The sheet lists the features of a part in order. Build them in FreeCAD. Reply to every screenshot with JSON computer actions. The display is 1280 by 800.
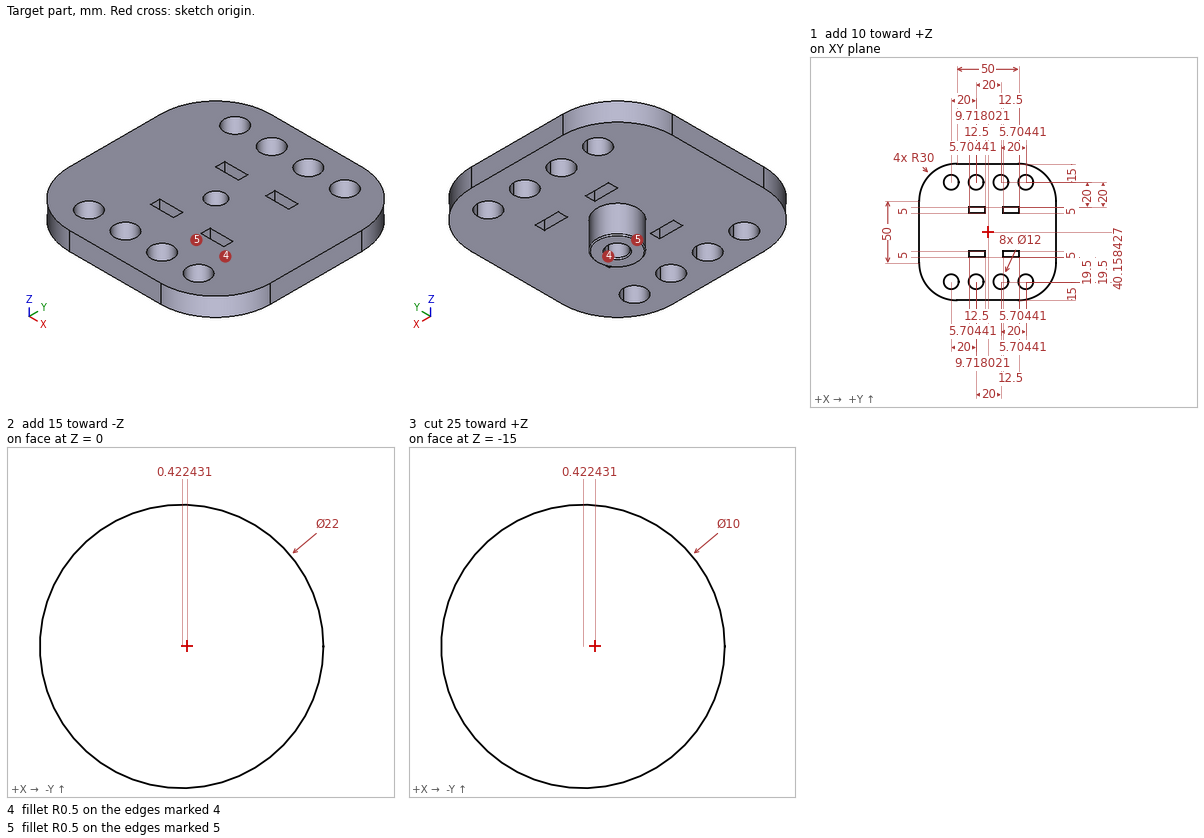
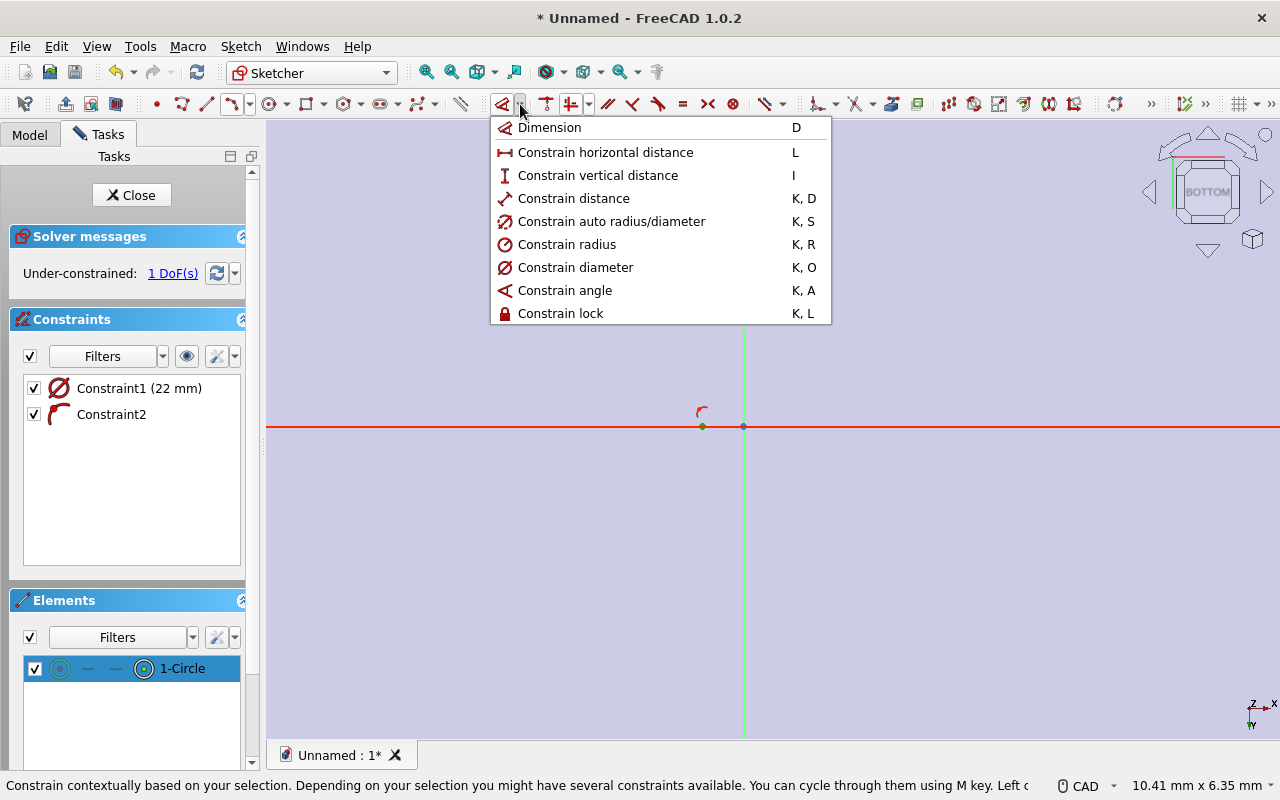
{"action": "left_click", "coordinate": [661, 152]}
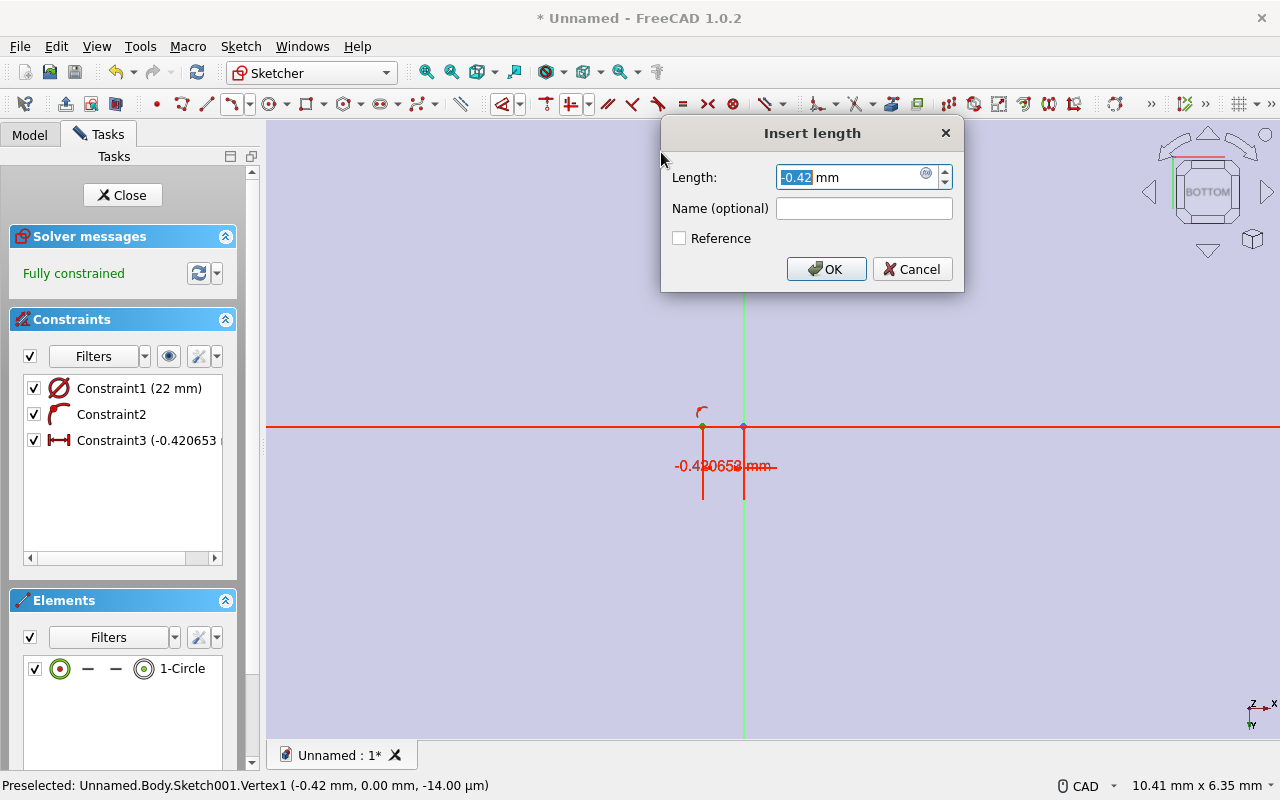
{"action": "type", "text": "-0.422431"}
{"action": "key", "text": "Return"}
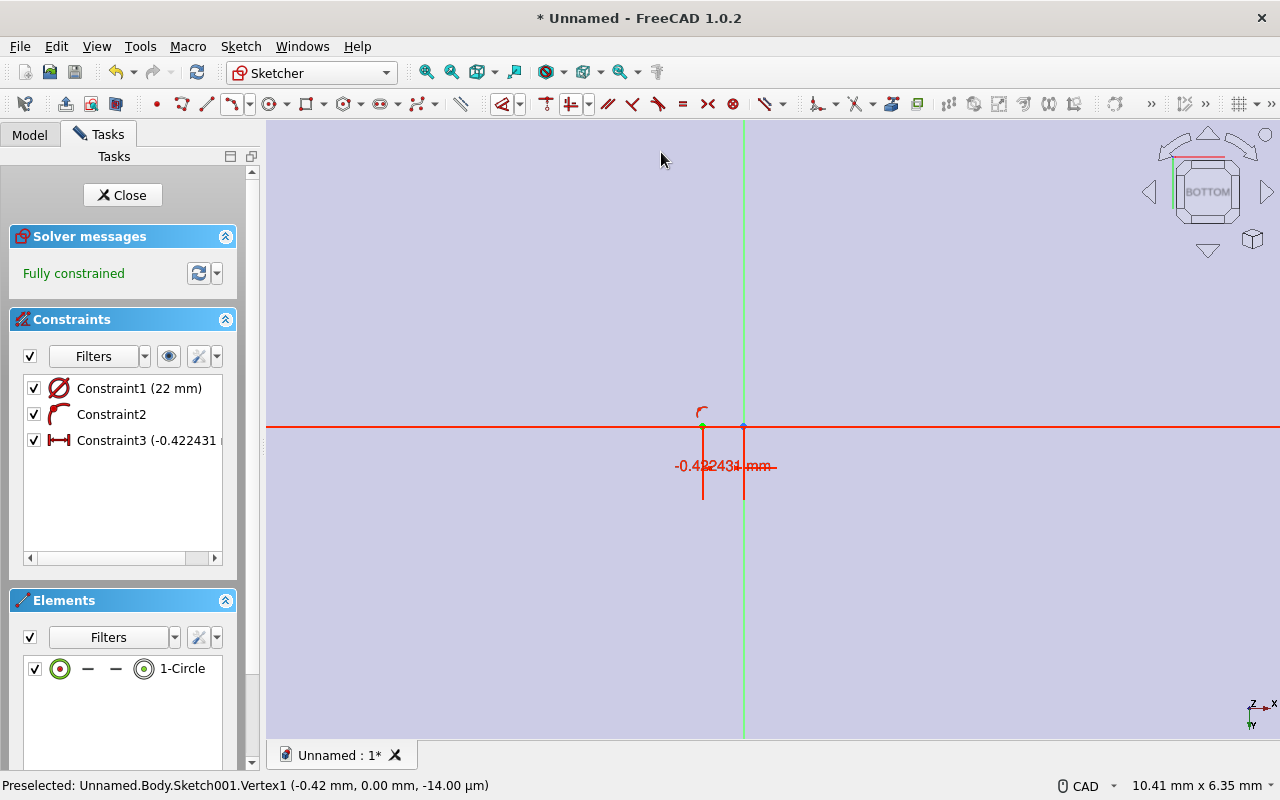
{"action": "left_click", "coordinate": [123, 195]}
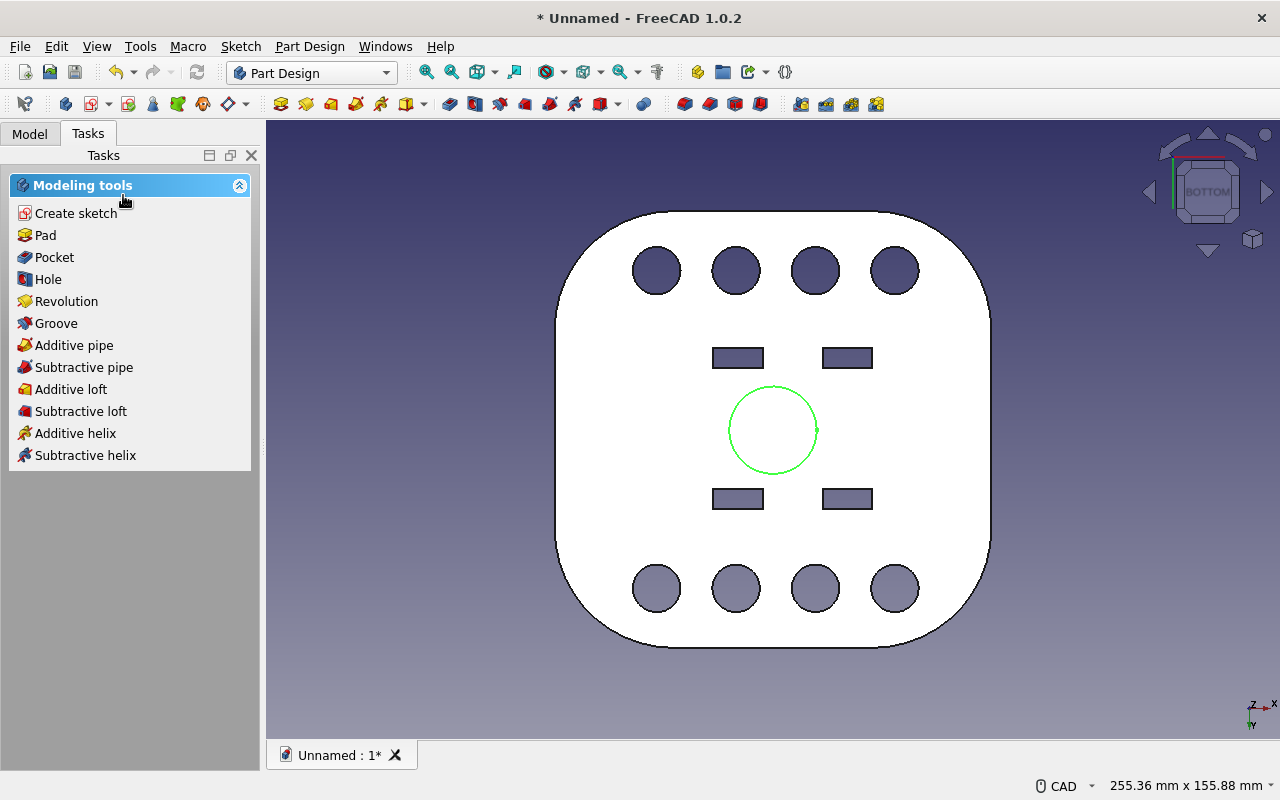
{"action": "left_click", "coordinate": [281, 104]}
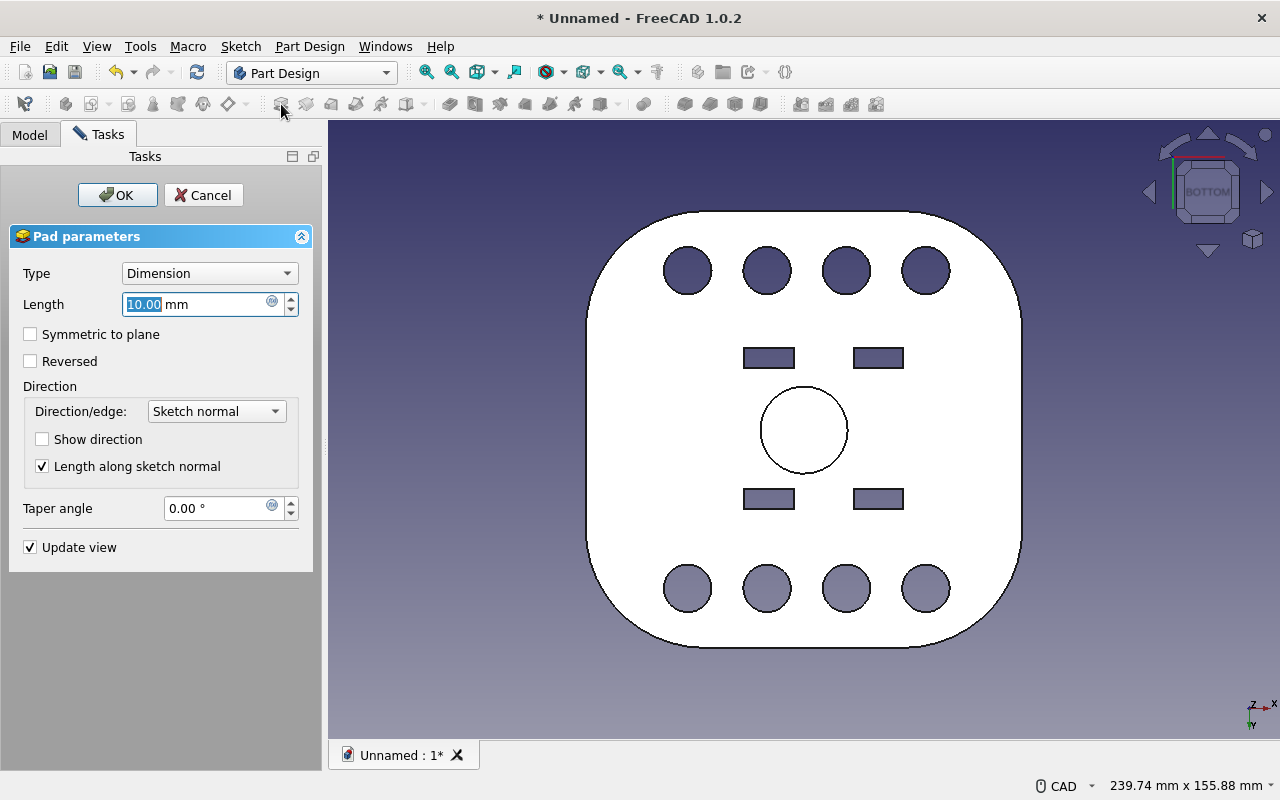
{"action": "type", "text": "15"}
{"action": "key", "text": "Tab"}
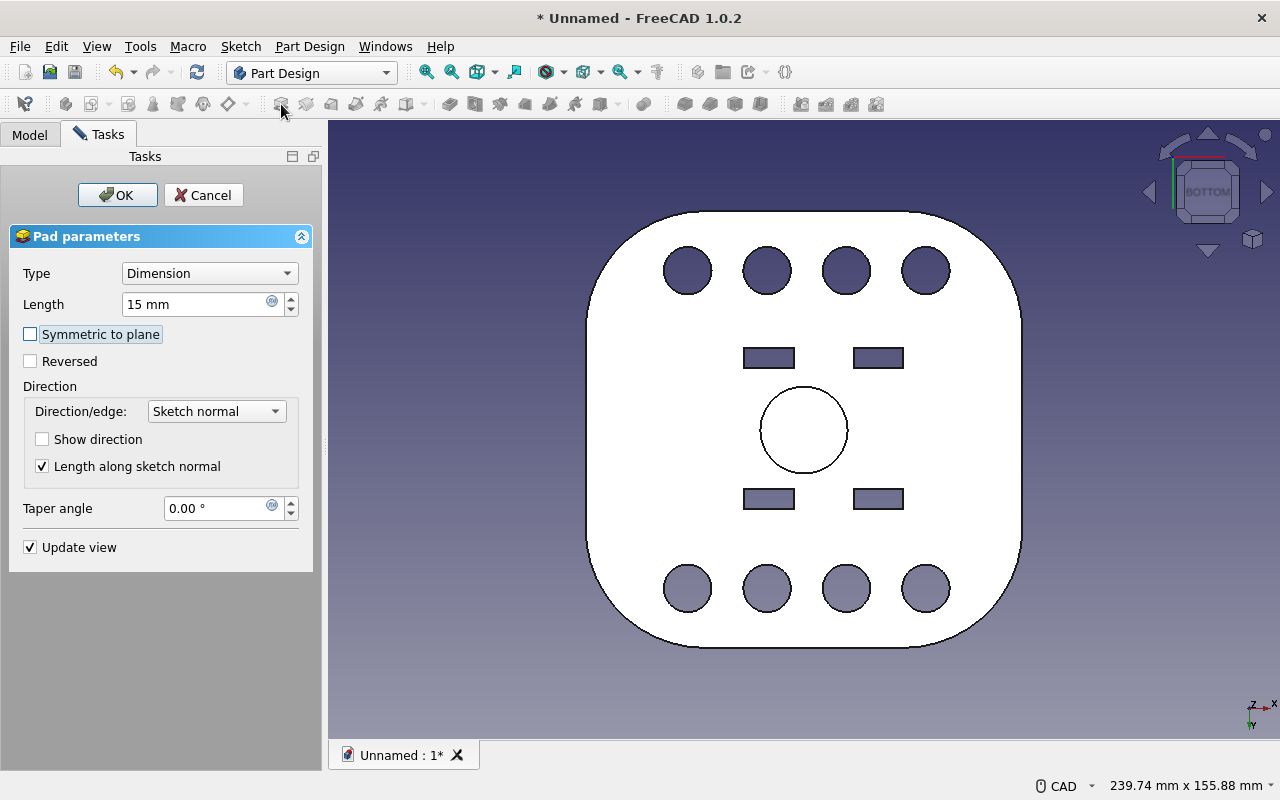
{"action": "left_click", "coordinate": [118, 195]}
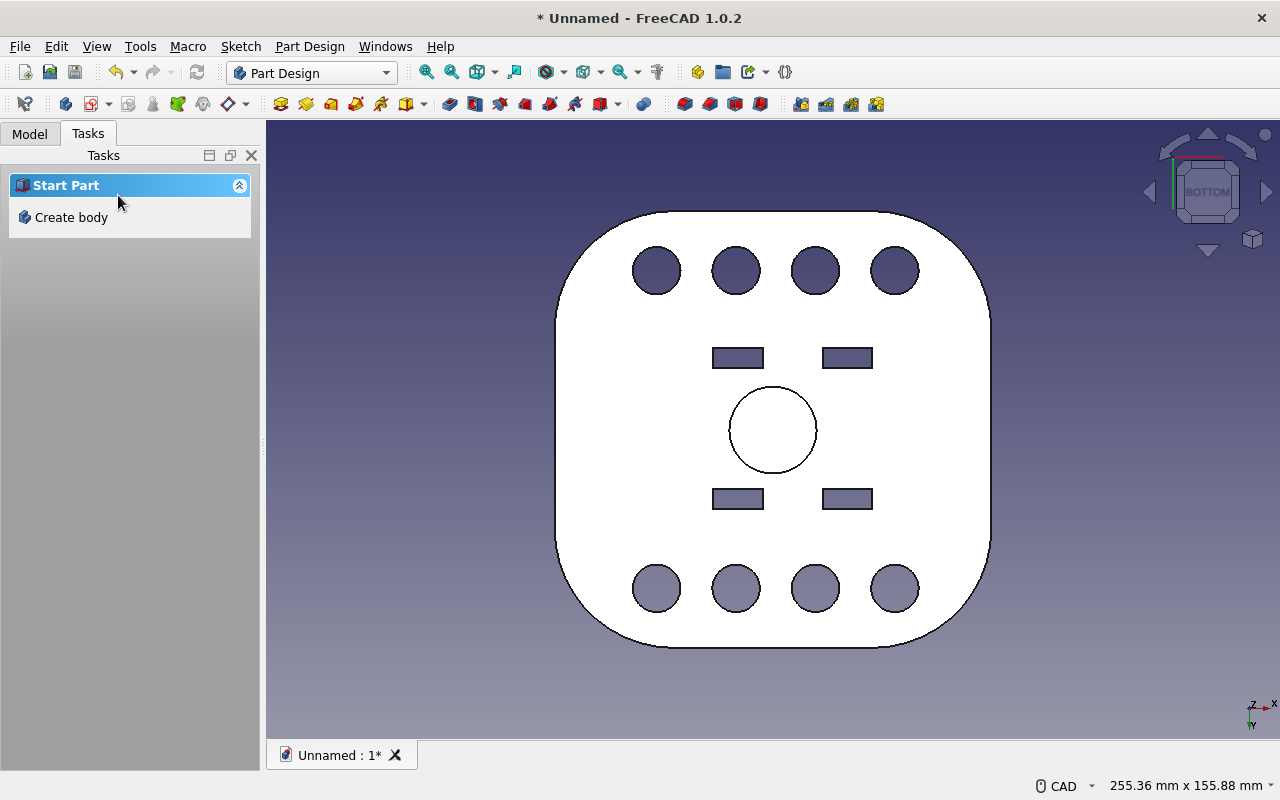
{"action": "left_click", "coordinate": [773, 429]}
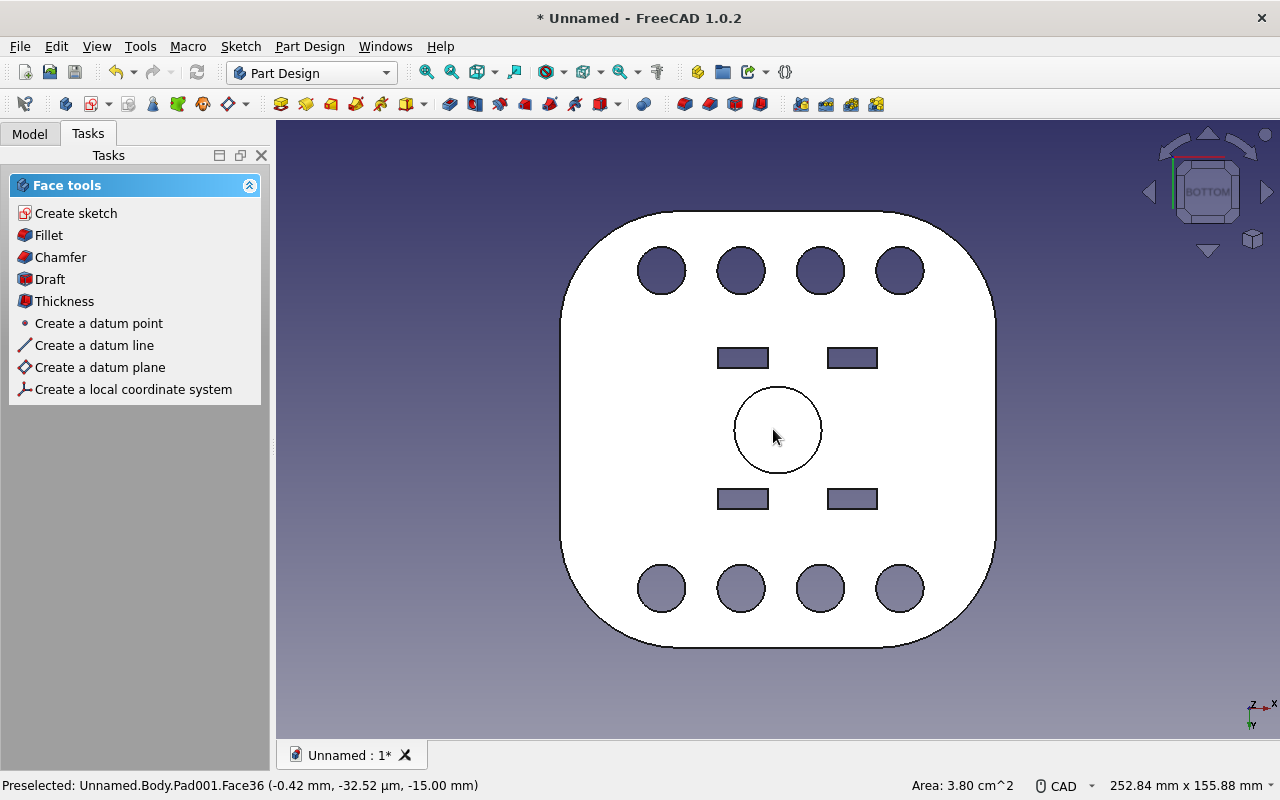
{"action": "left_click", "coordinate": [90, 104]}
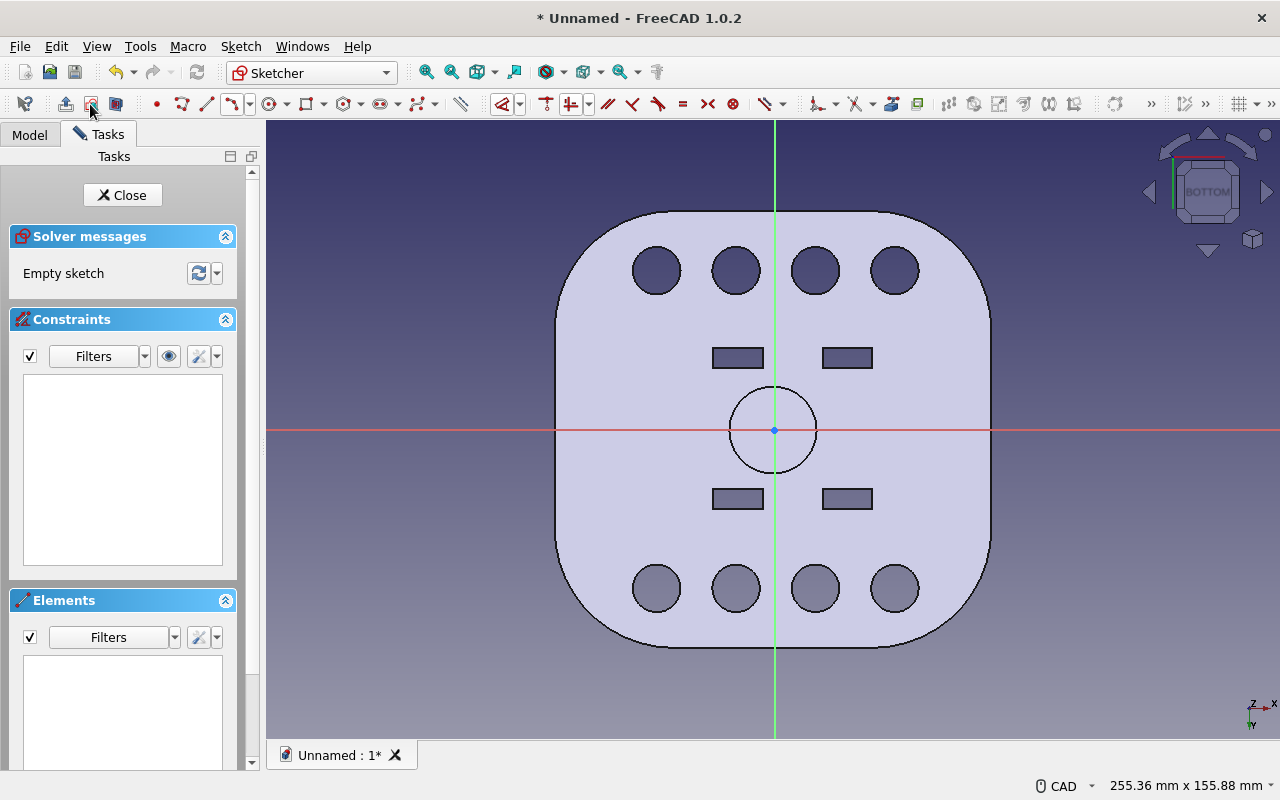
{"action": "scroll", "coordinate": [780, 430], "scroll_direction": "up", "scroll_amount": 12}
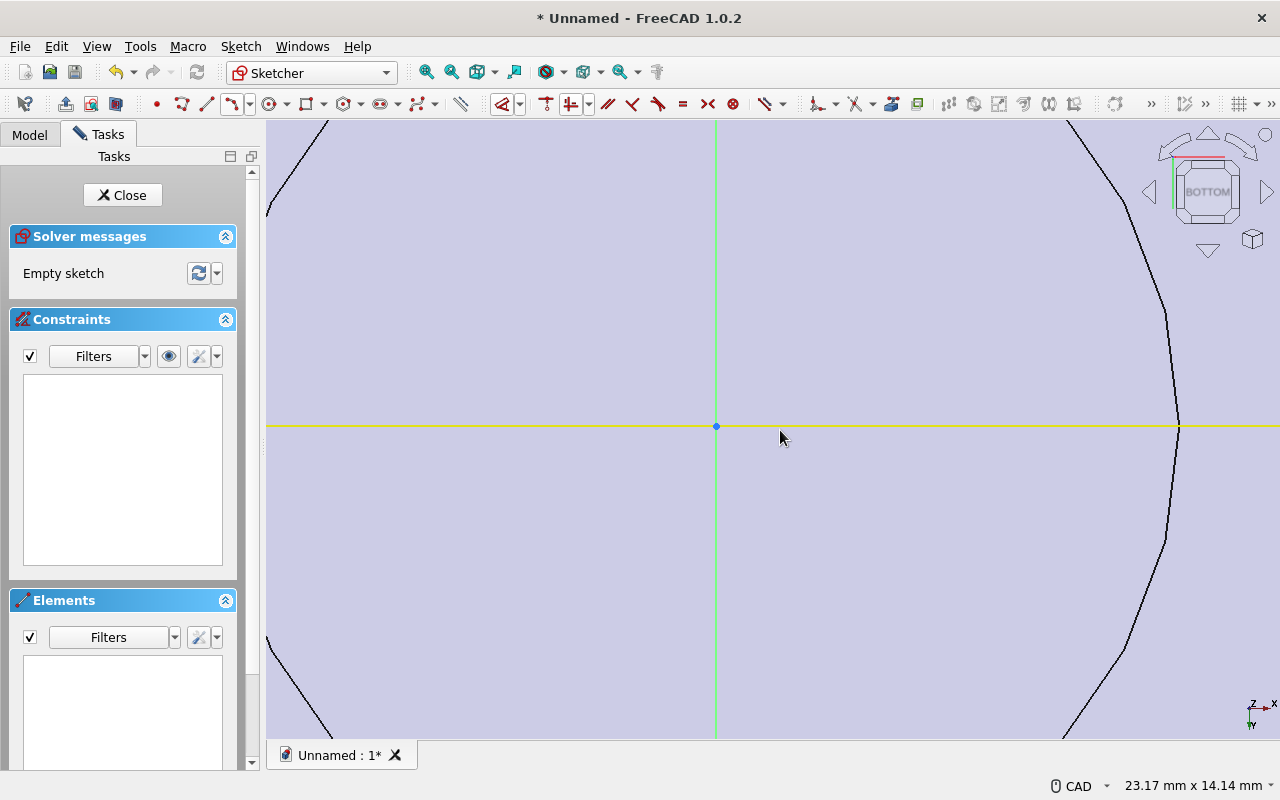
{"action": "left_click", "coordinate": [268, 104]}